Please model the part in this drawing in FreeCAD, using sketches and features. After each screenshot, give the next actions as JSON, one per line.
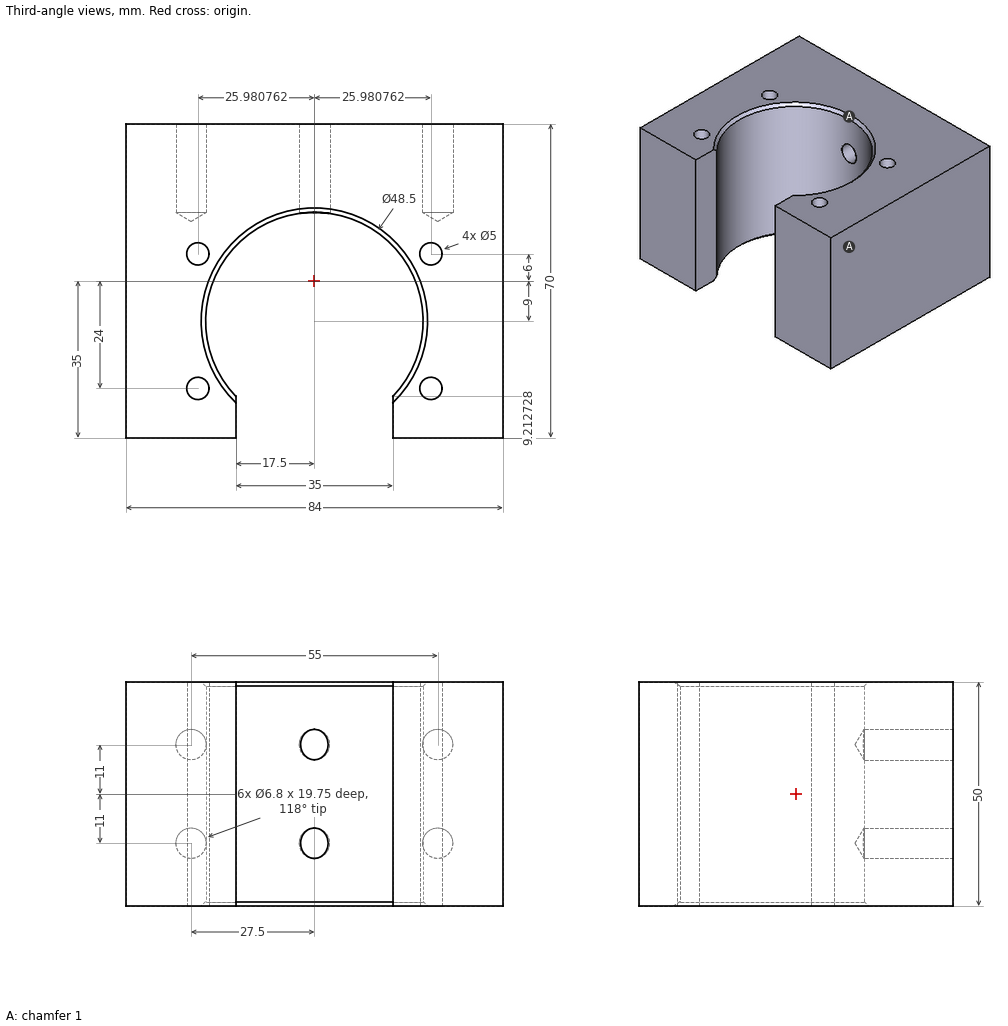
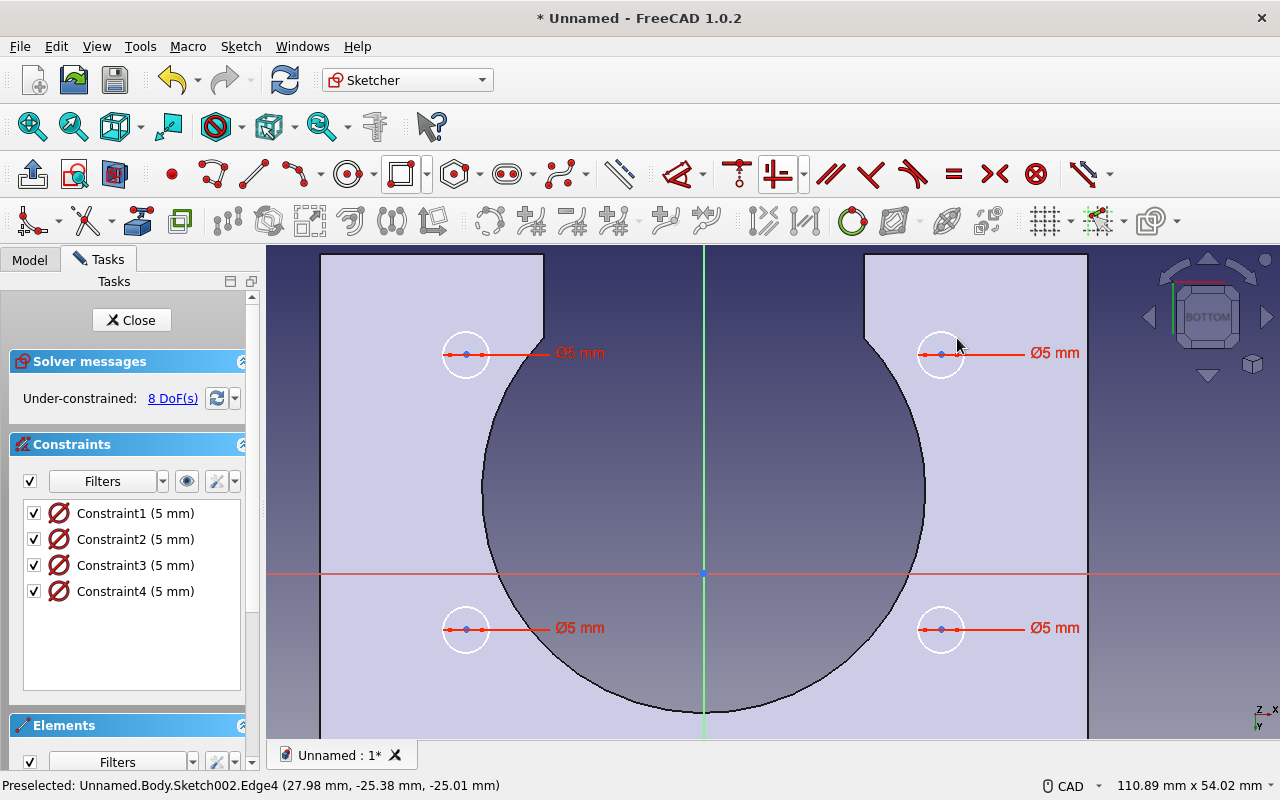
{"action": "left_click", "coordinate": [941, 630]}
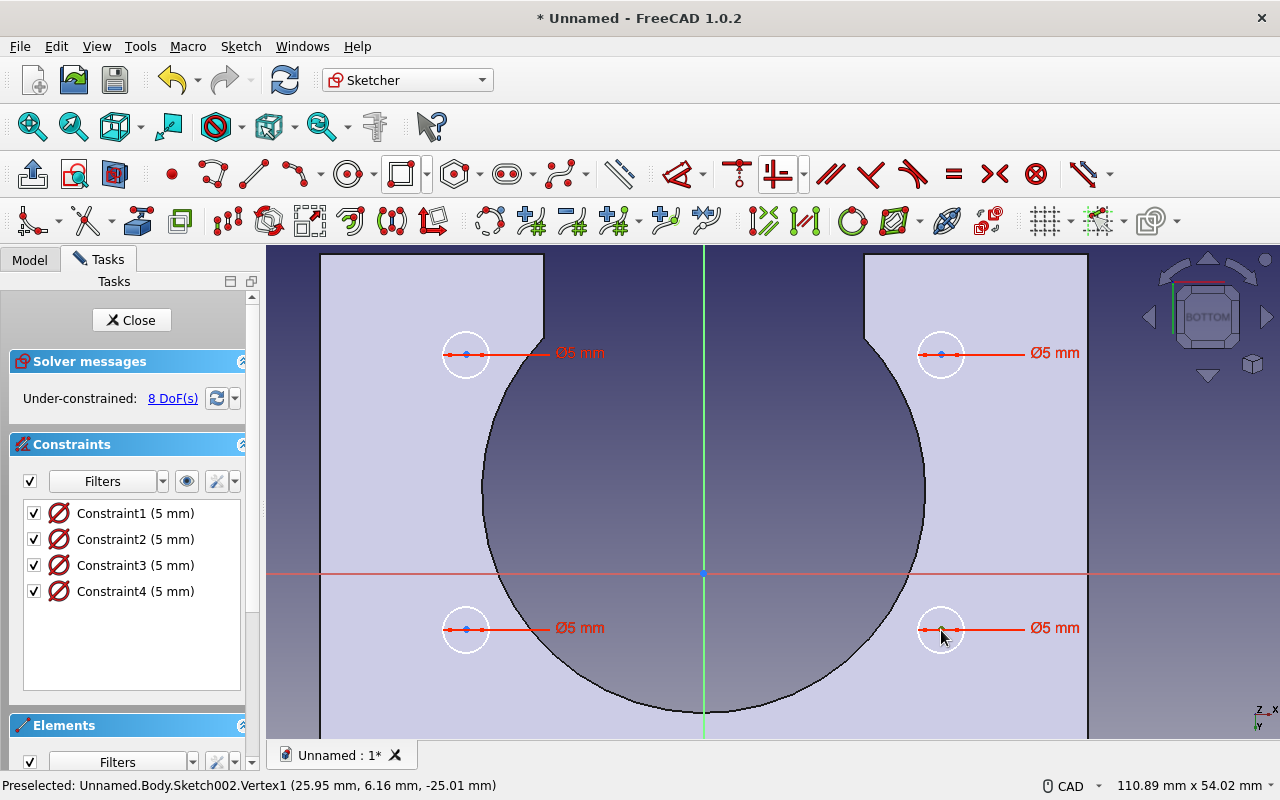
{"action": "left_click", "coordinate": [466, 630]}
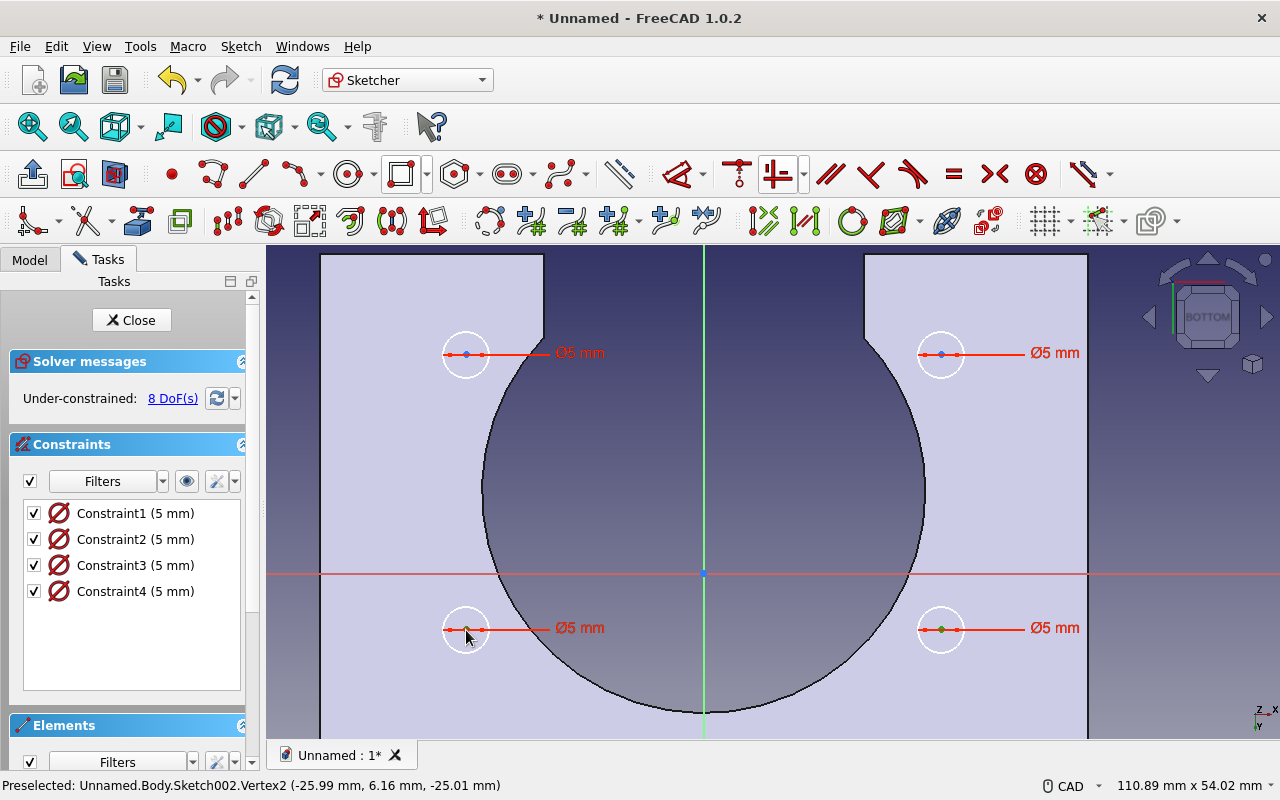
{"action": "key", "text": "h"}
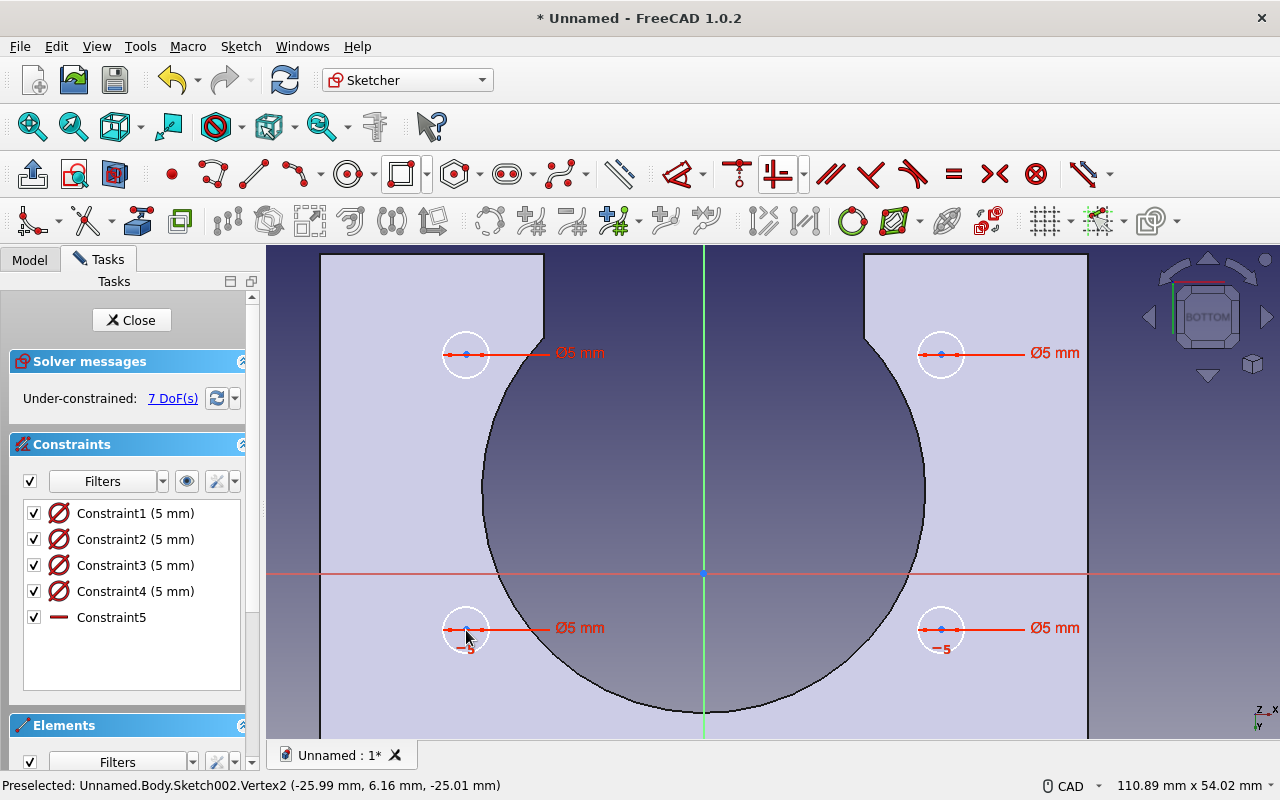
{"action": "left_click", "coordinate": [466, 630]}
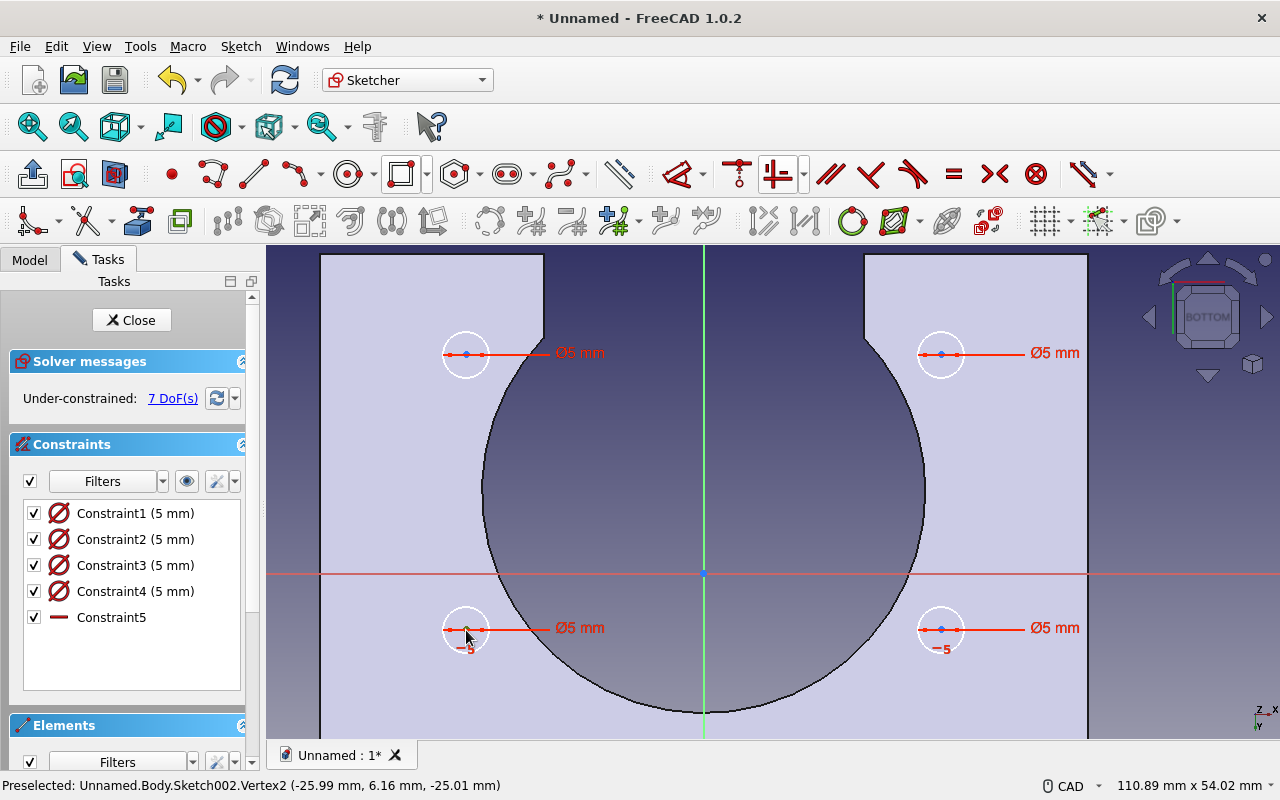
{"action": "left_click", "coordinate": [466, 355]}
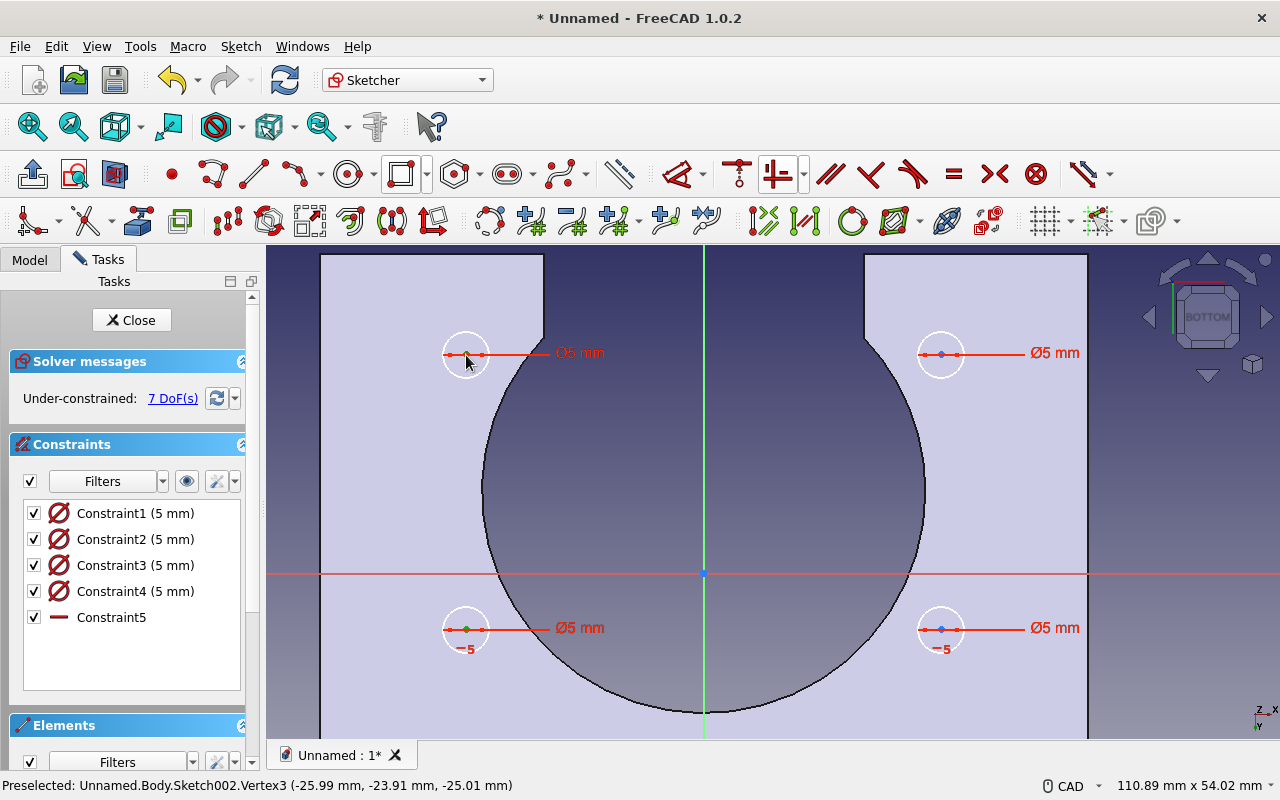
{"action": "left_click", "coordinate": [804, 174]}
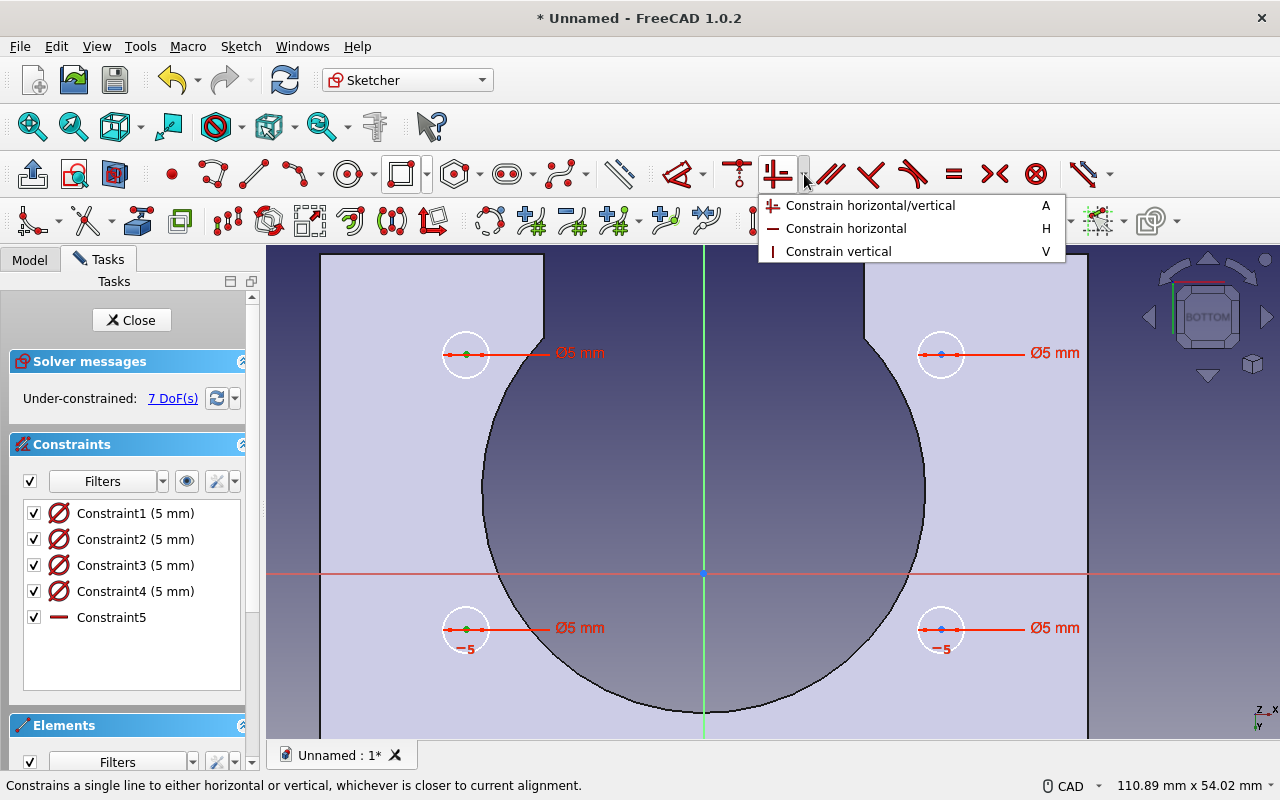
{"action": "left_click", "coordinate": [912, 252]}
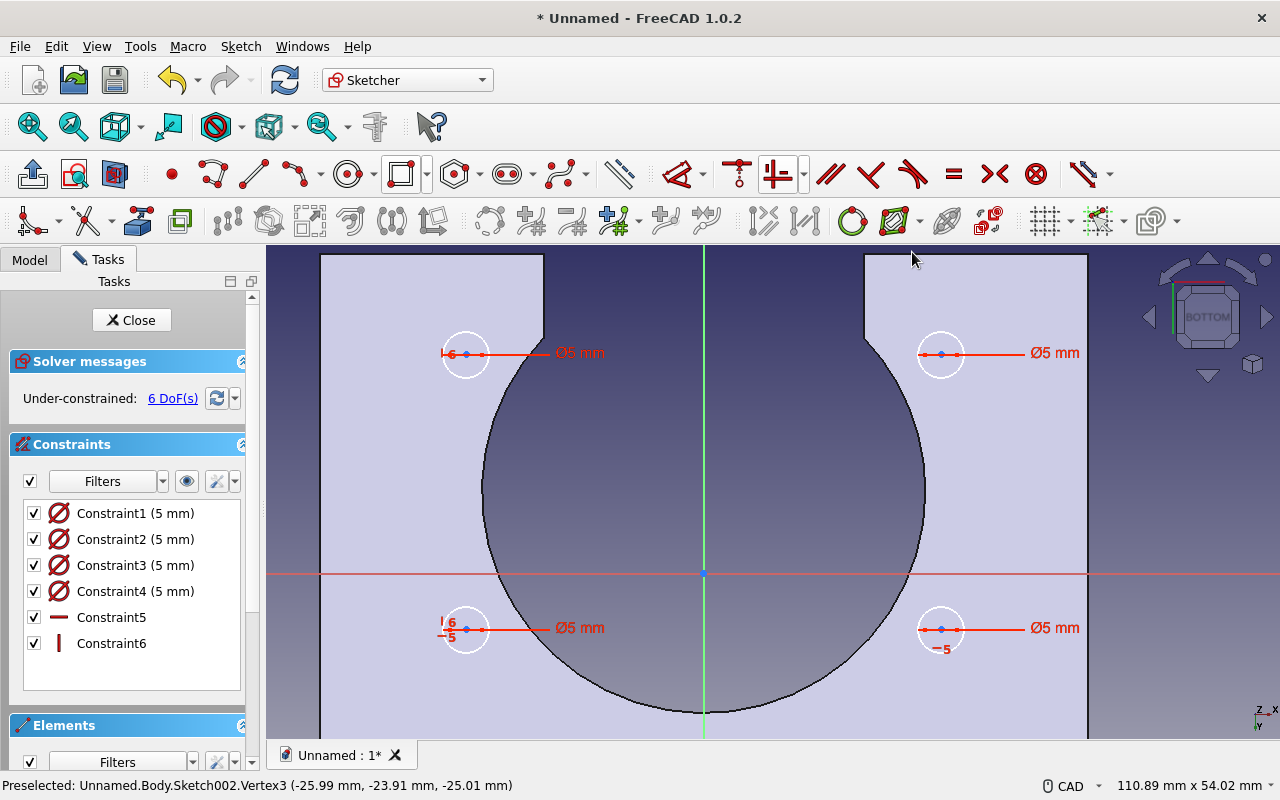
{"action": "left_click", "coordinate": [941, 630]}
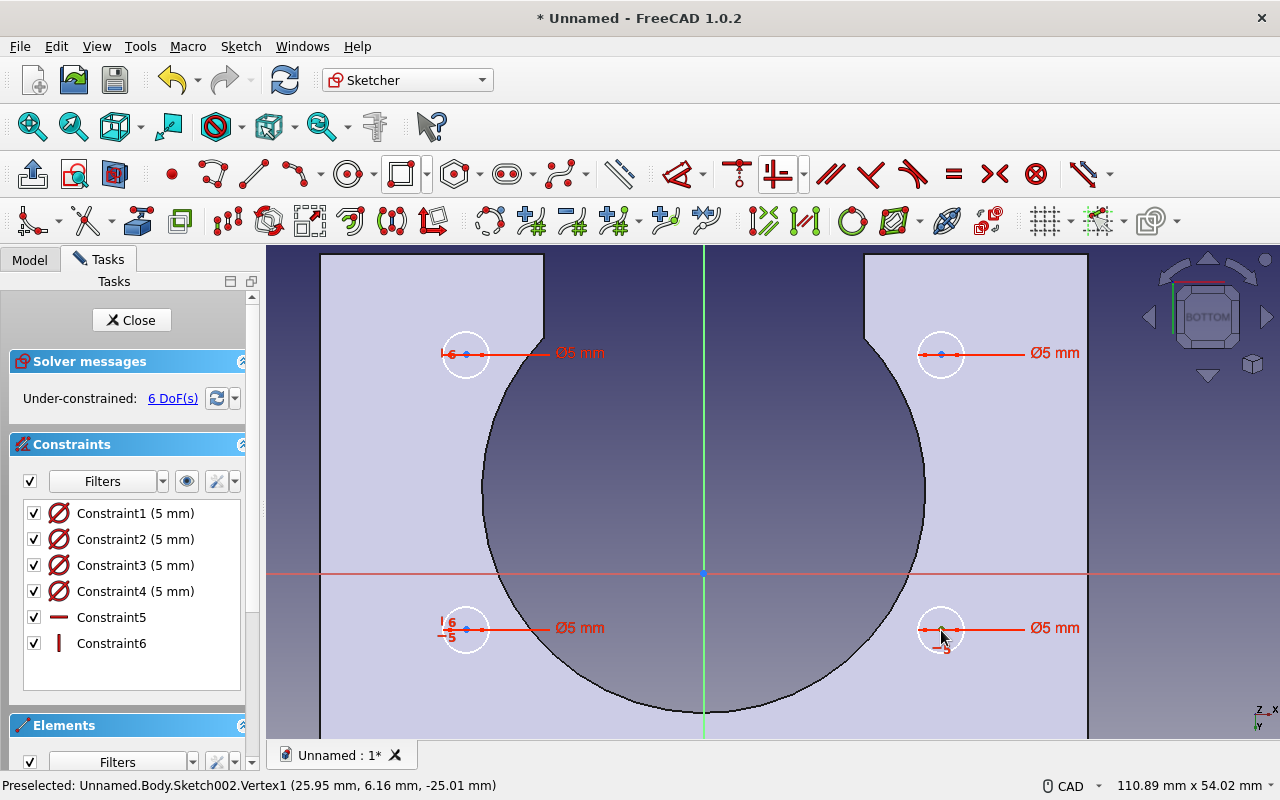
{"action": "left_click", "coordinate": [941, 355]}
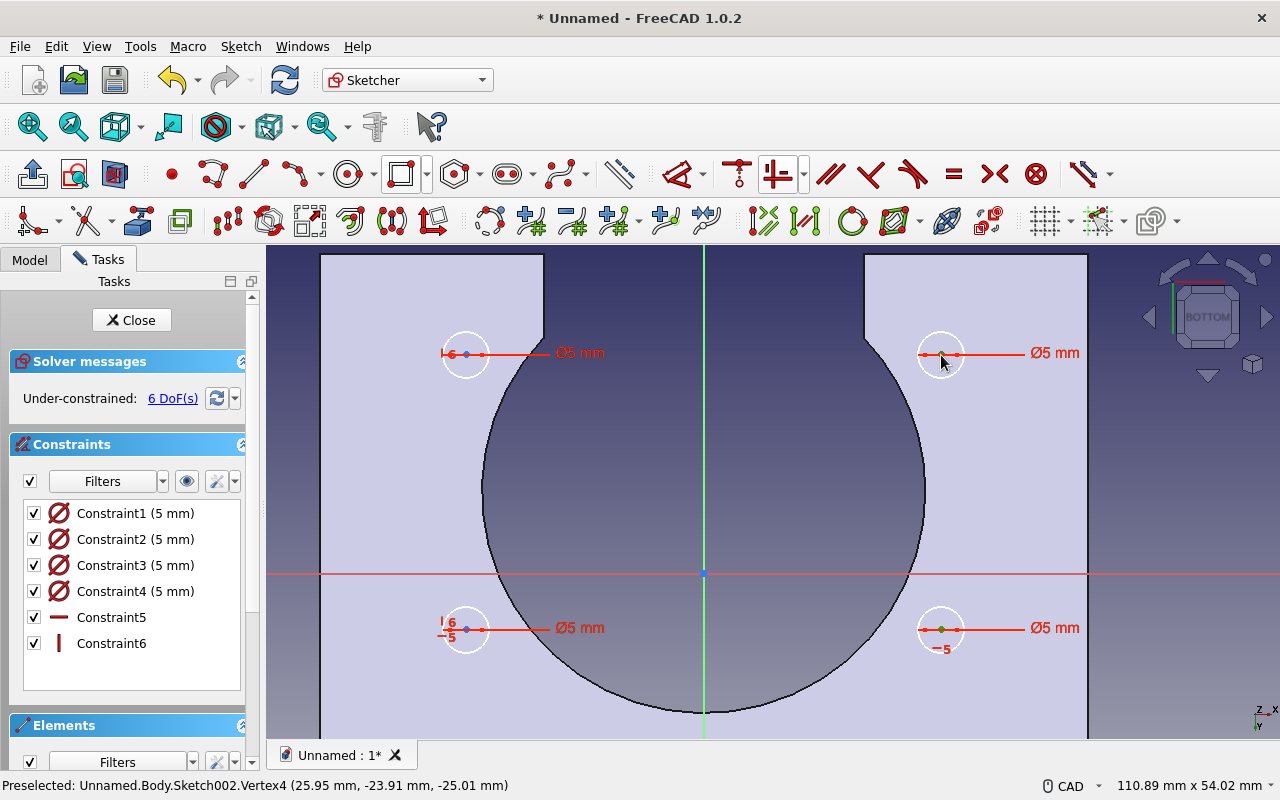
{"action": "key", "text": "v"}